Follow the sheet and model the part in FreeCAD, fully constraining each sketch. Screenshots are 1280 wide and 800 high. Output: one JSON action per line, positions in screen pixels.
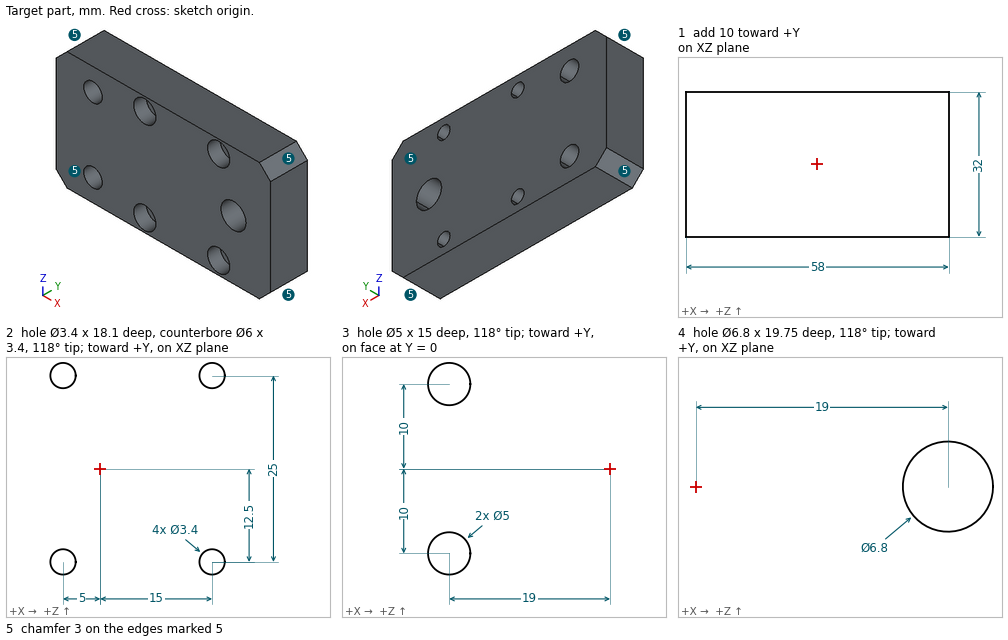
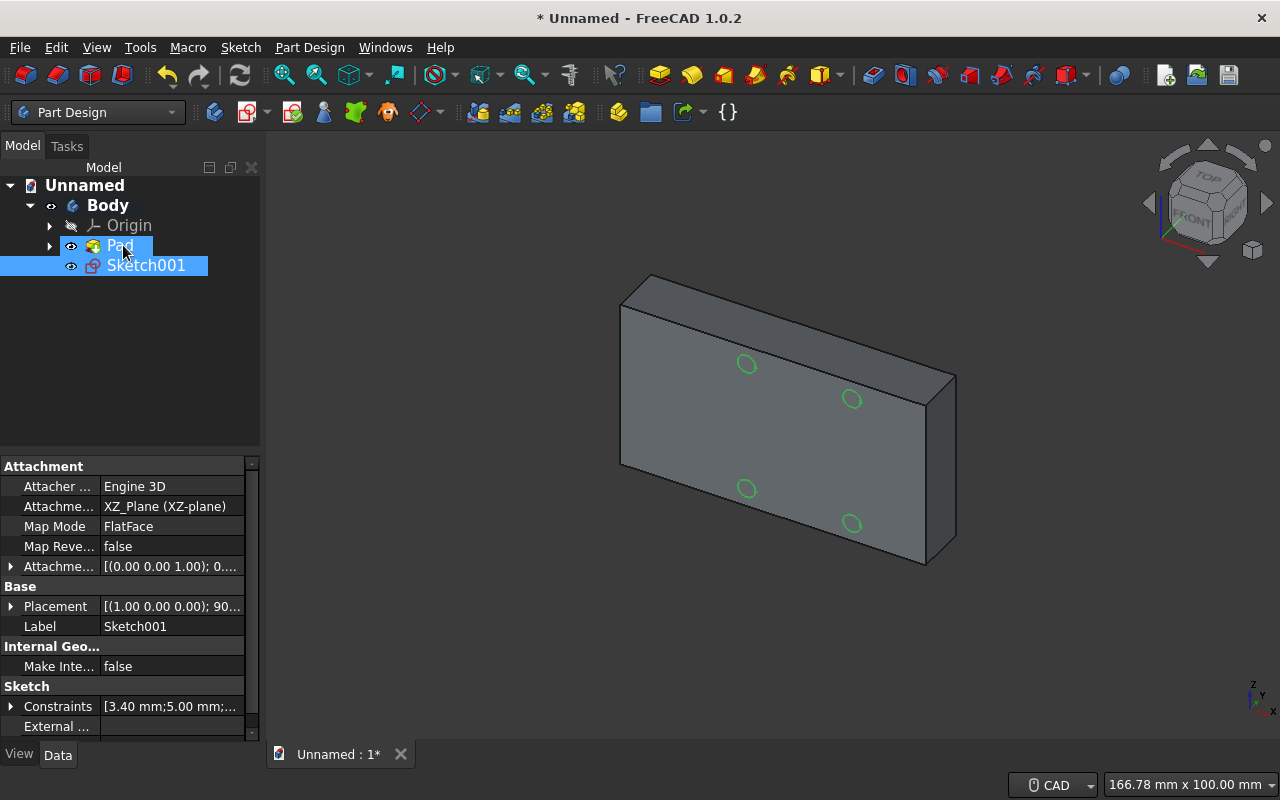
{"action": "left_click", "coordinate": [906, 76]}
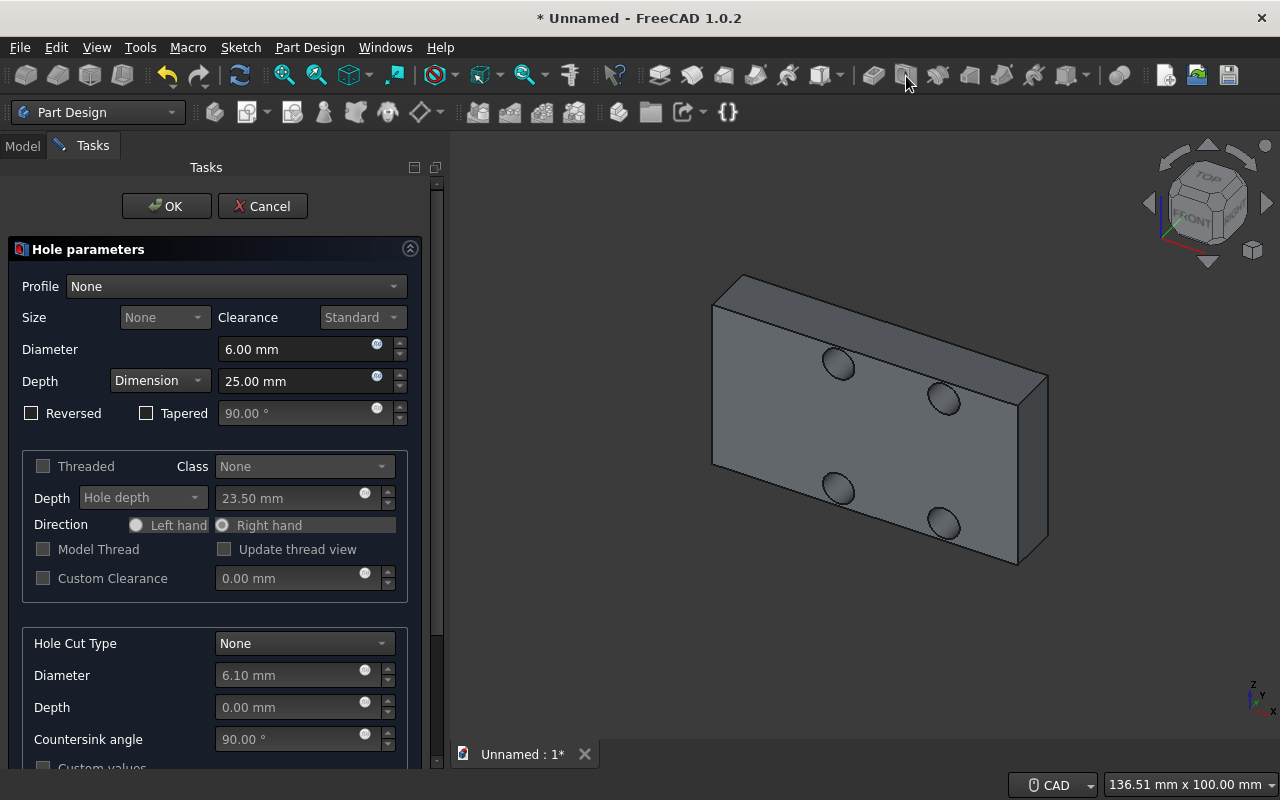
{"action": "triple_click", "coordinate": [305, 349]}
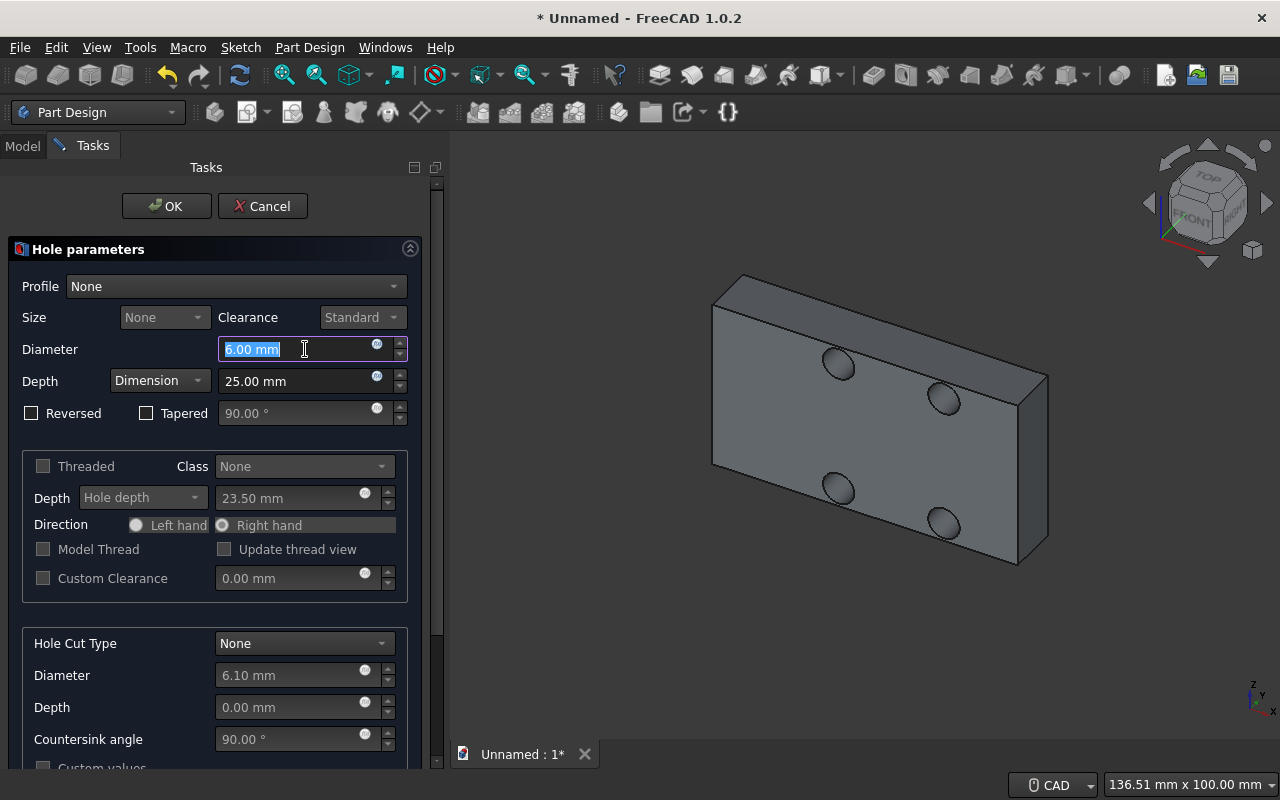
{"action": "type", "text": "3.4"}
{"action": "key", "text": "Tab"}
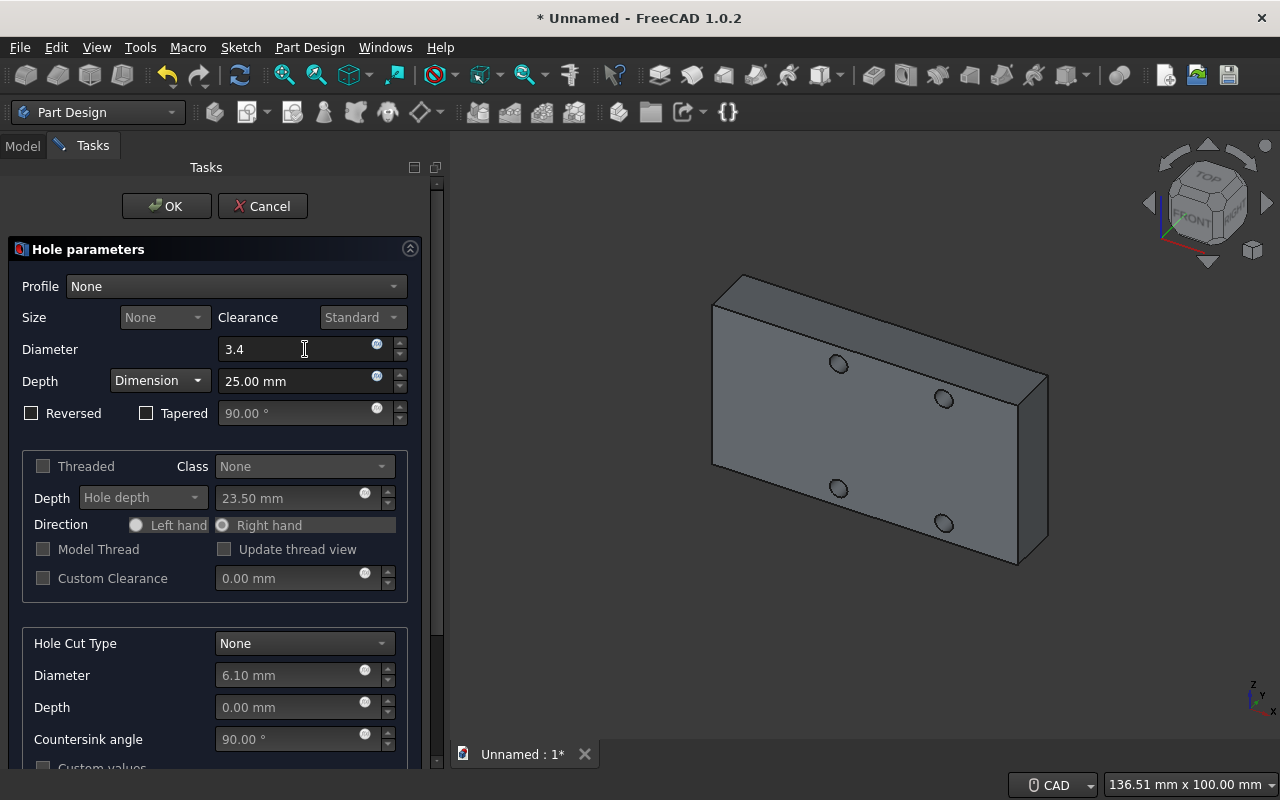
{"action": "triple_click", "coordinate": [305, 381]}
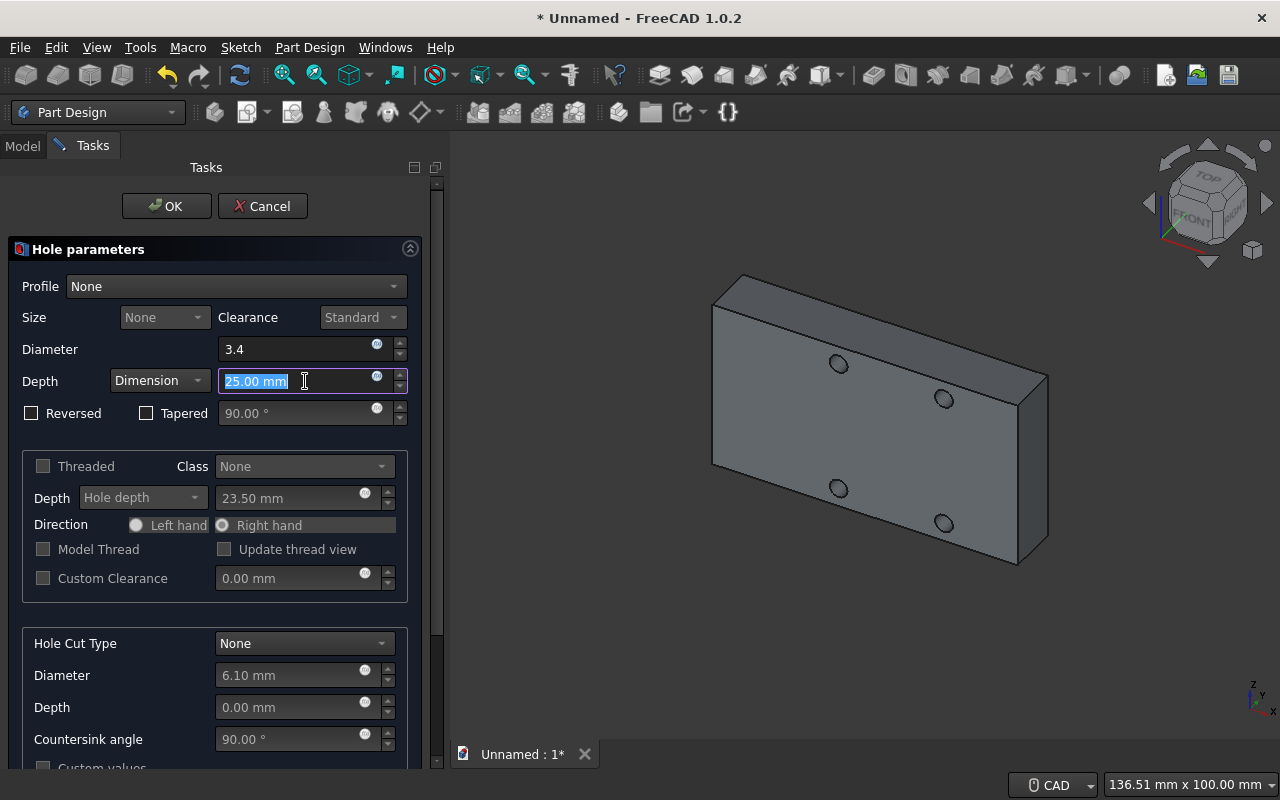
{"action": "type", "text": "18.1"}
{"action": "key", "text": "Tab"}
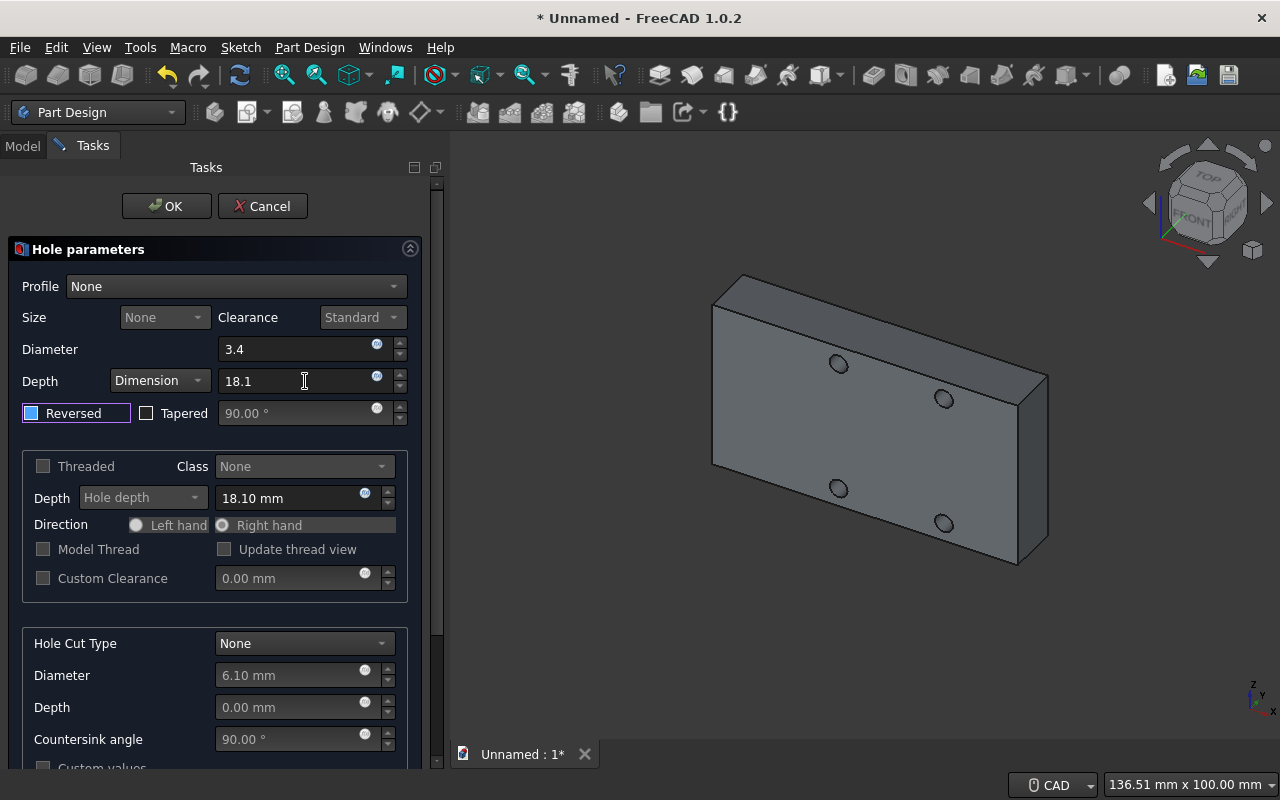
{"action": "left_click", "coordinate": [306, 644]}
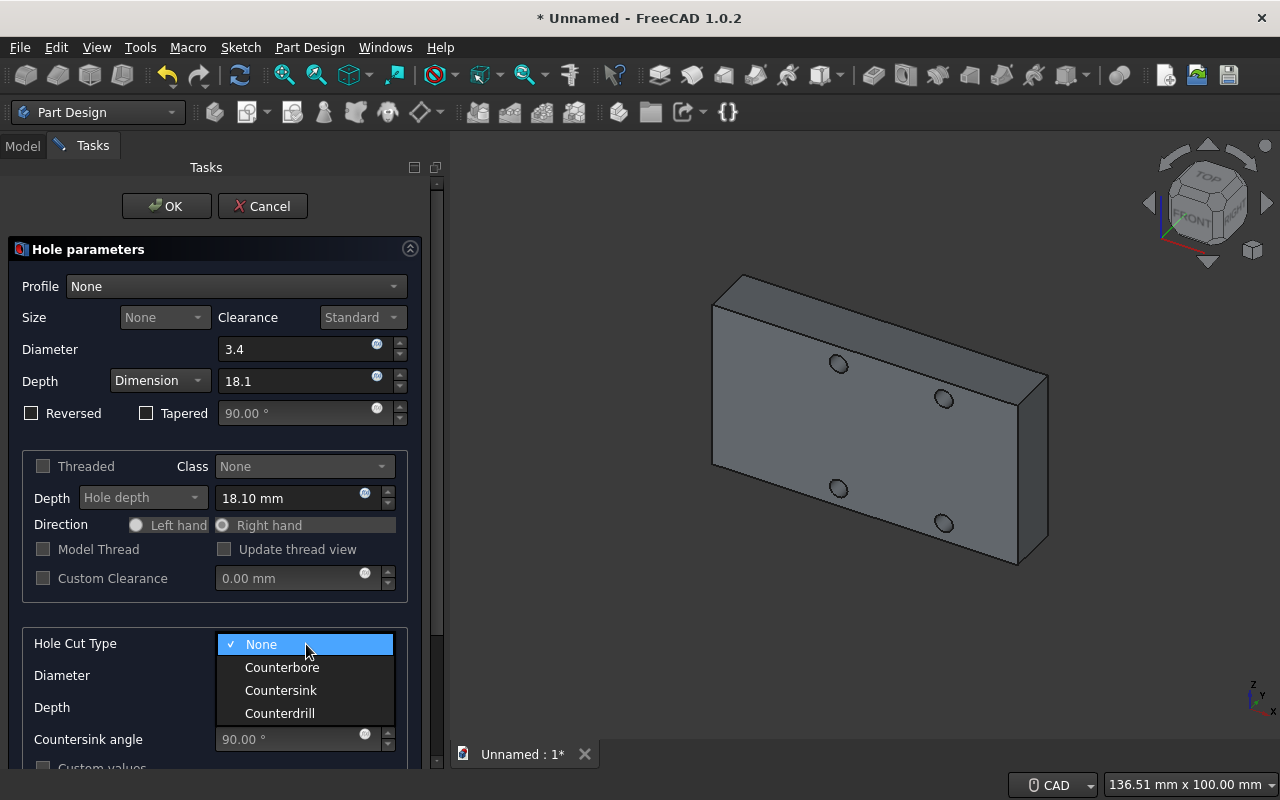
{"action": "left_click", "coordinate": [304, 668]}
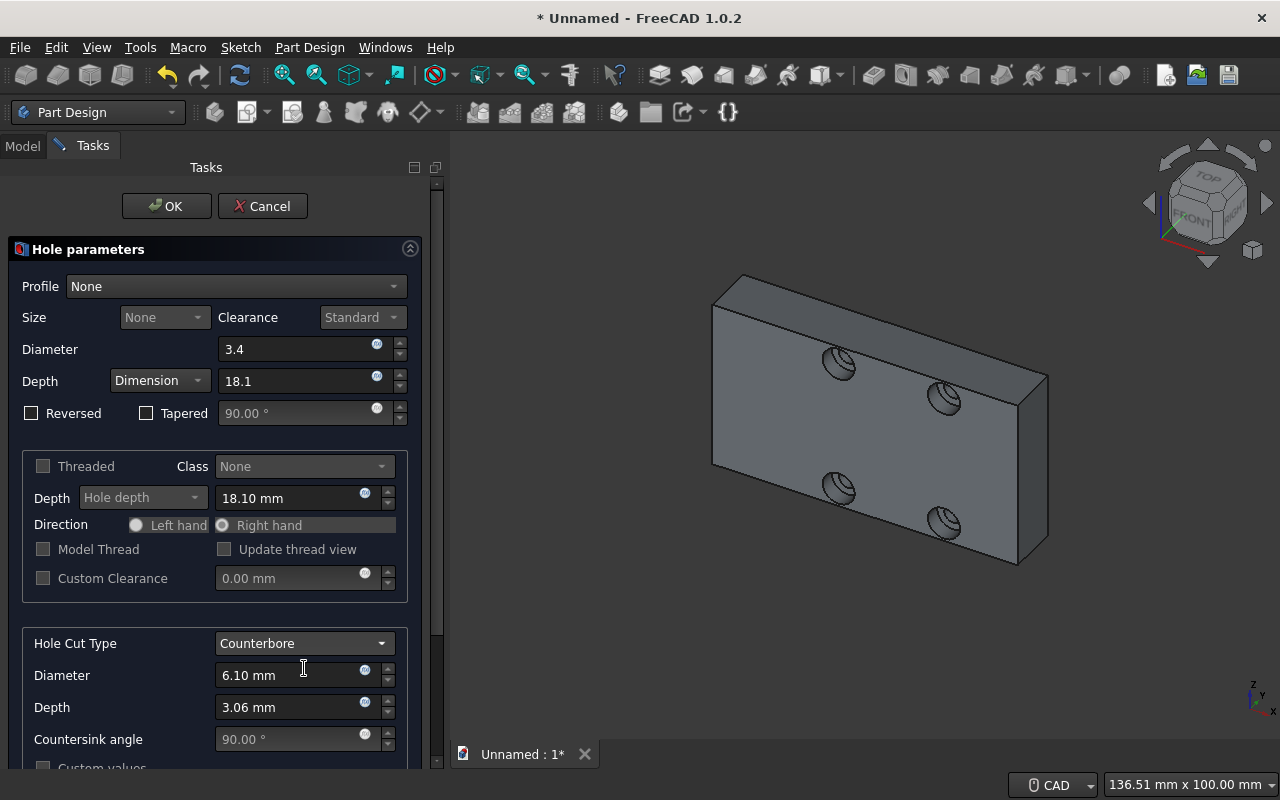
{"action": "triple_click", "coordinate": [298, 675]}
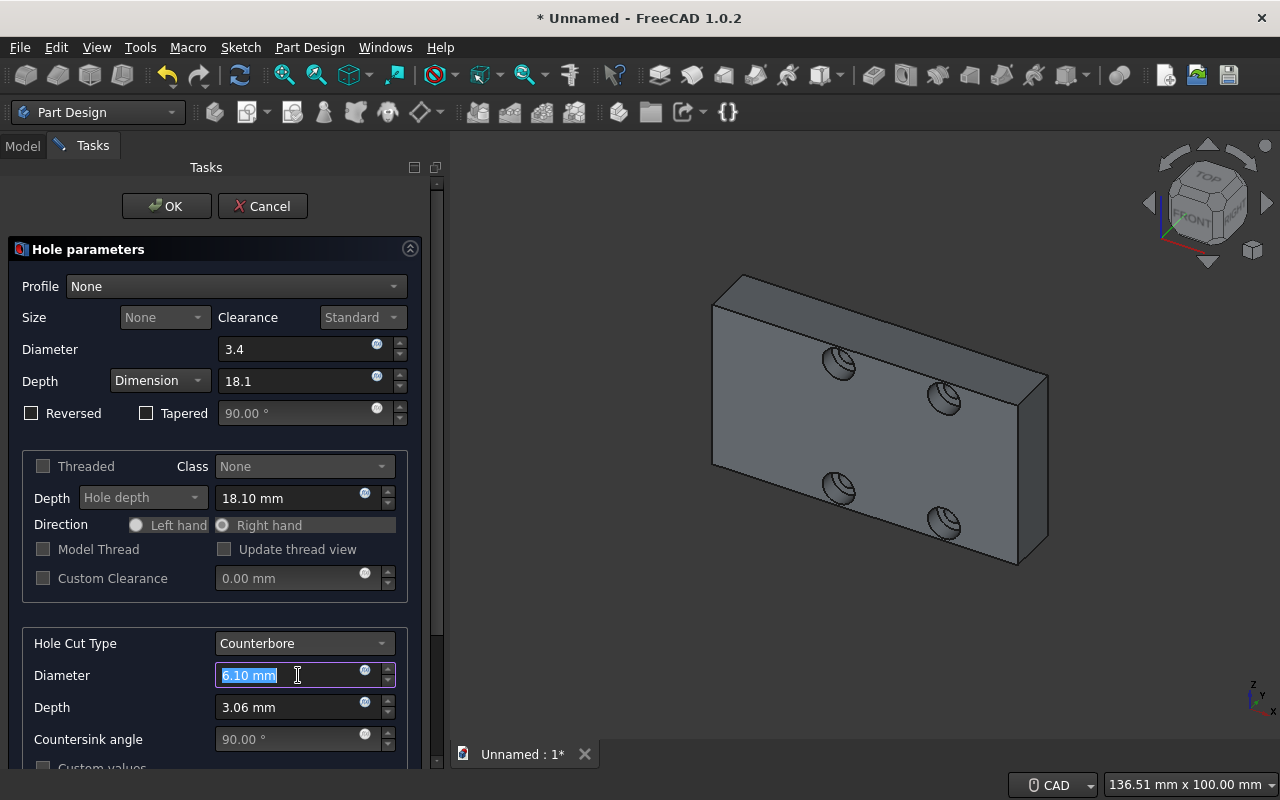
{"action": "type", "text": "6"}
{"action": "key", "text": "Tab"}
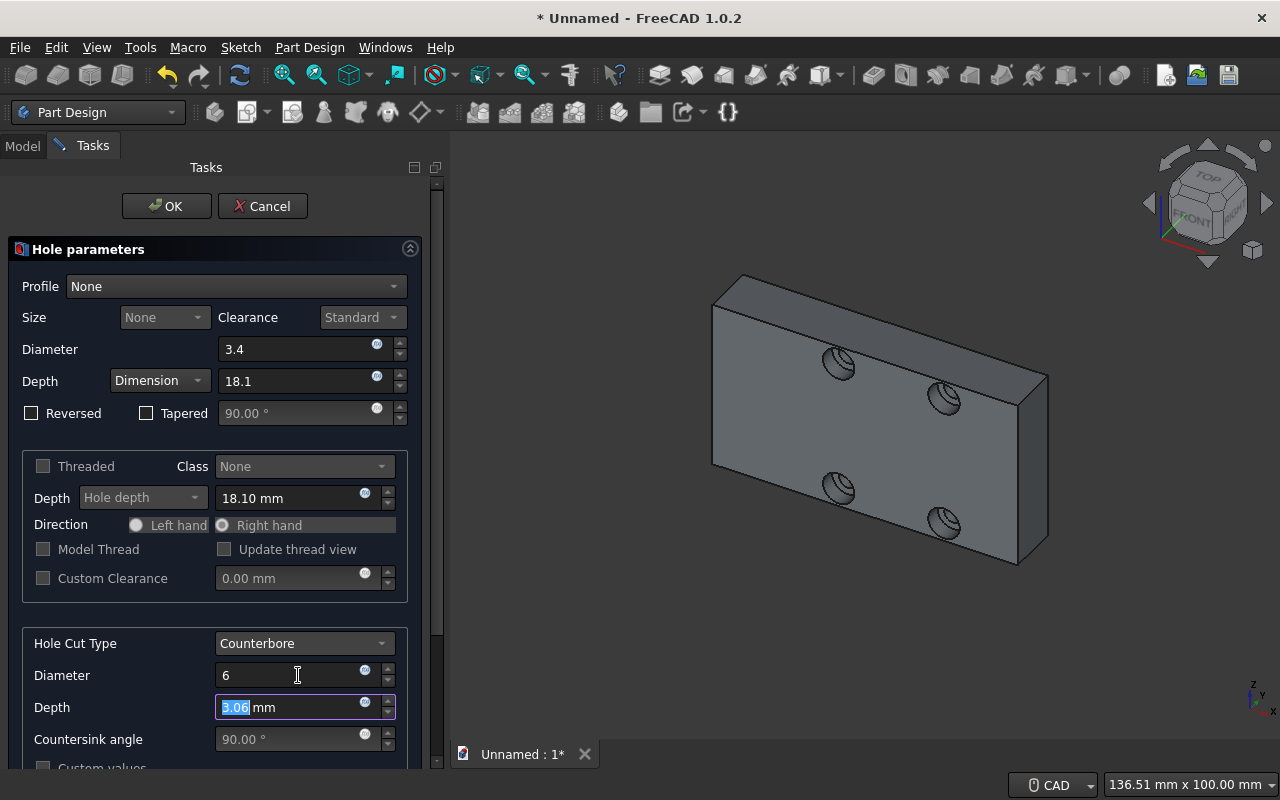
{"action": "type", "text": "3.4"}
{"action": "key", "text": "Tab"}